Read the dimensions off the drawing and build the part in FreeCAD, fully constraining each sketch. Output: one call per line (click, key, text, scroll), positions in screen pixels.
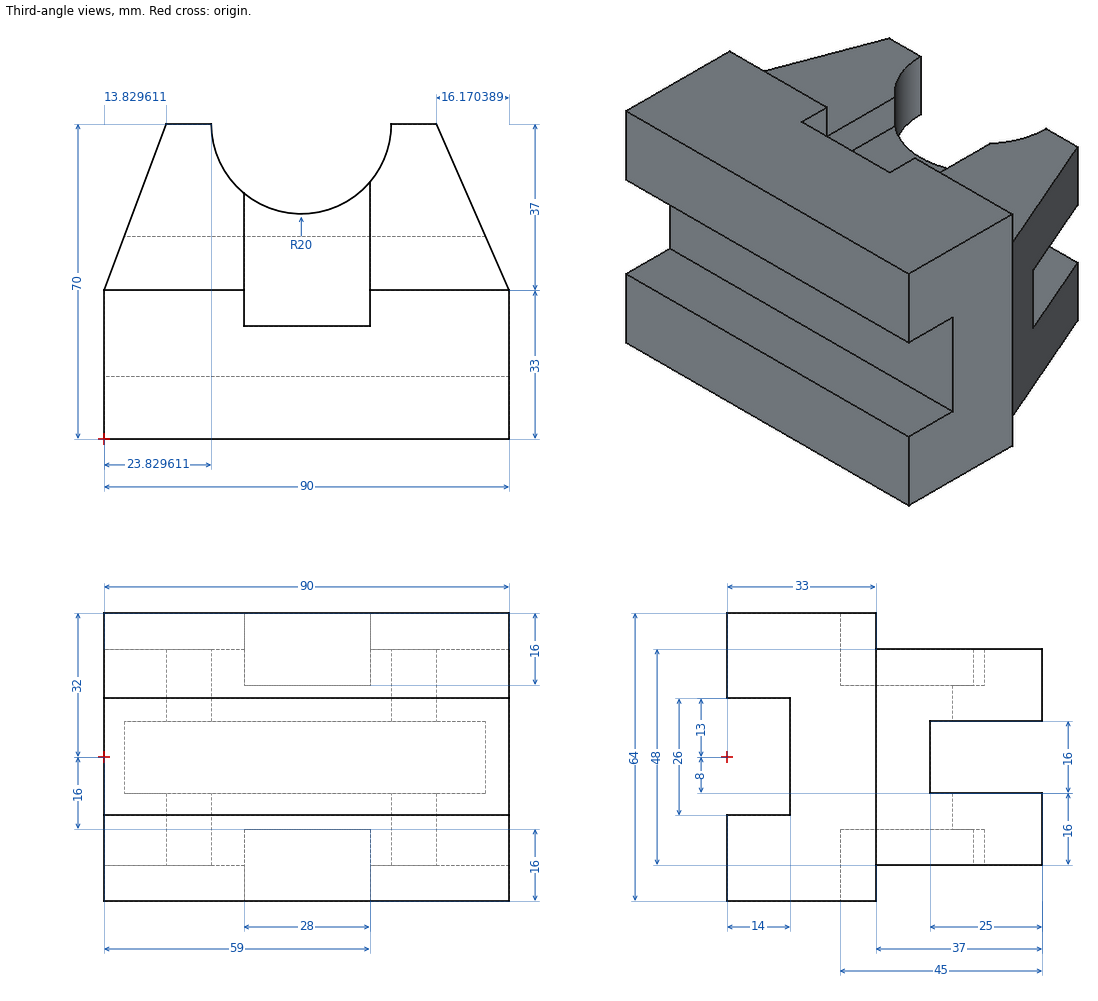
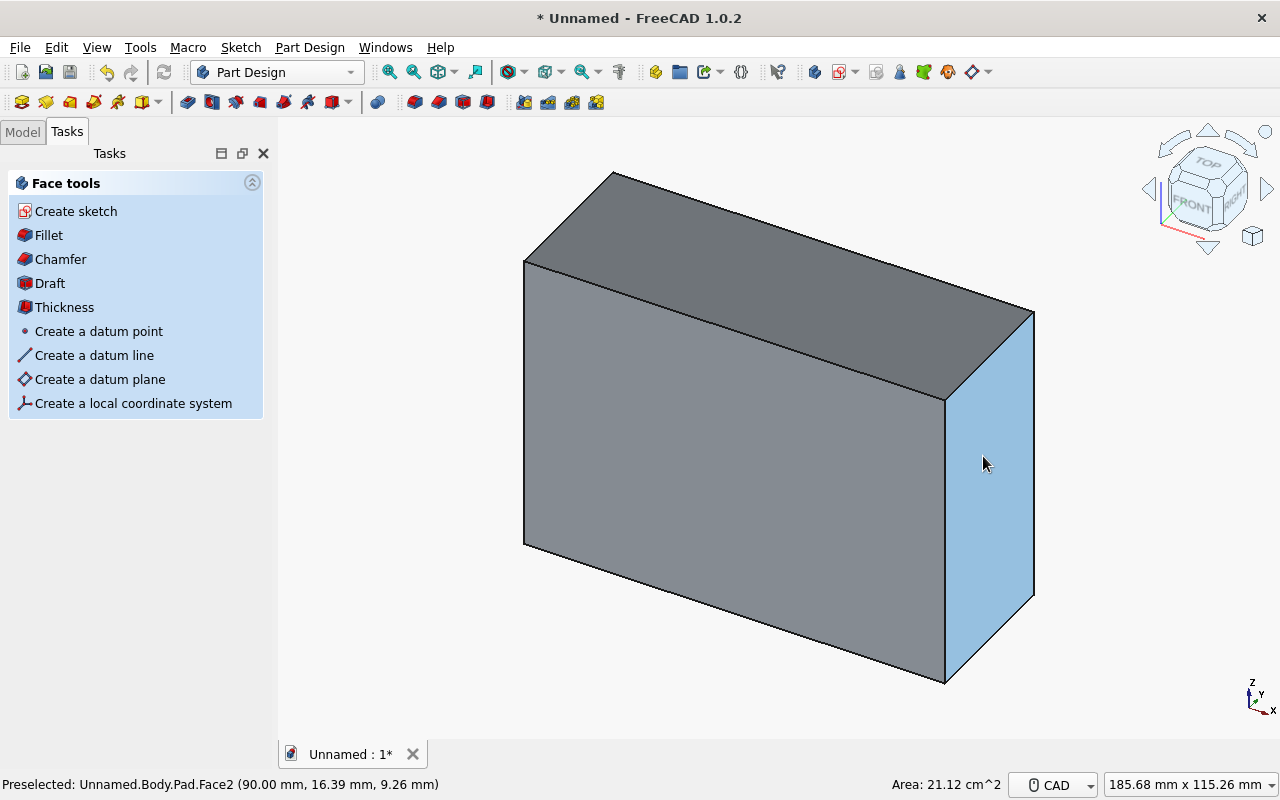
click(840, 72)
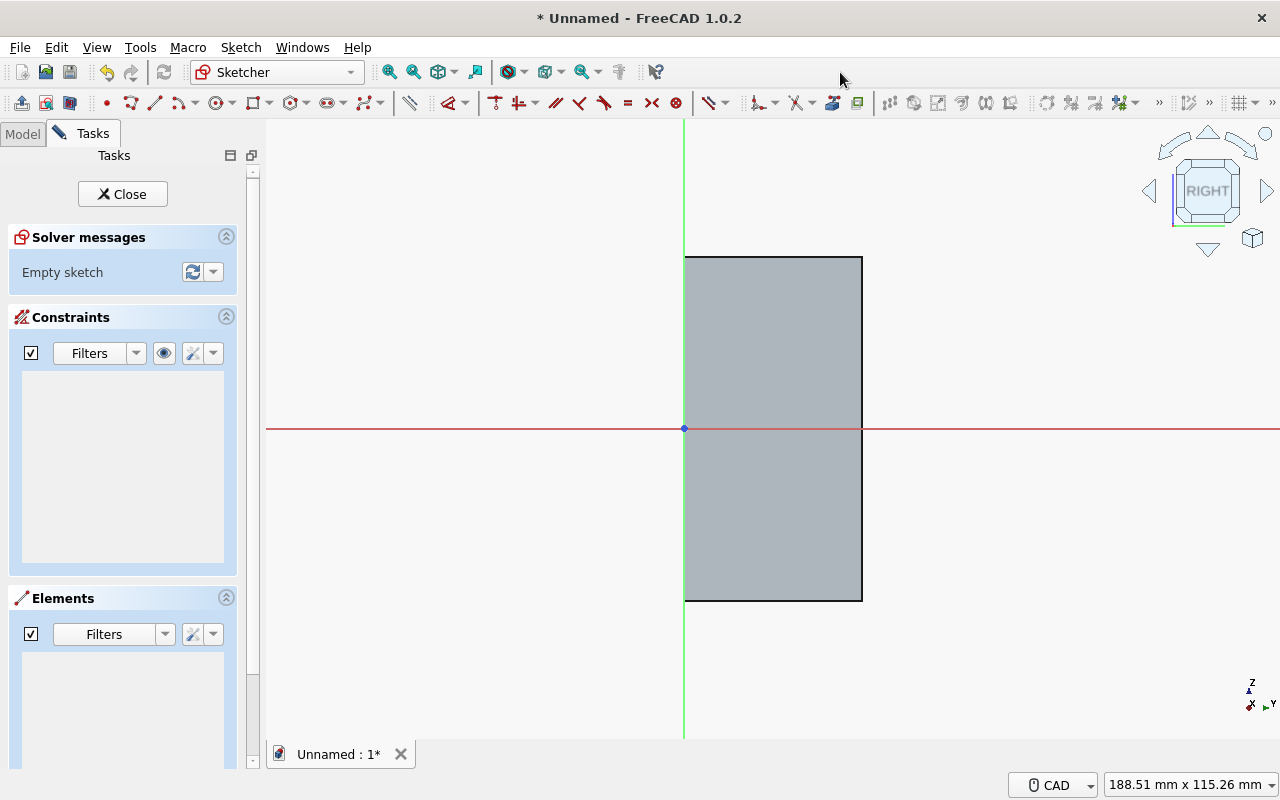
scroll(732, 429, up, 5)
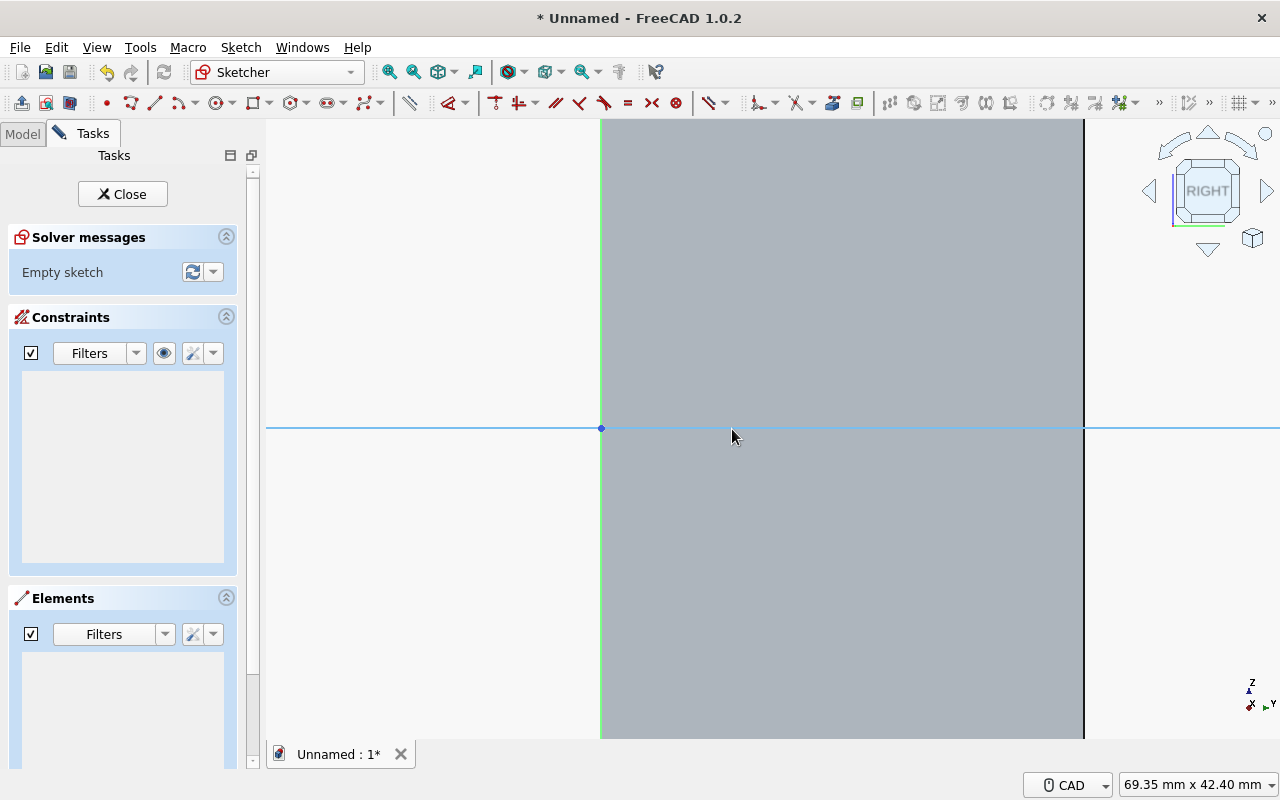
click(254, 104)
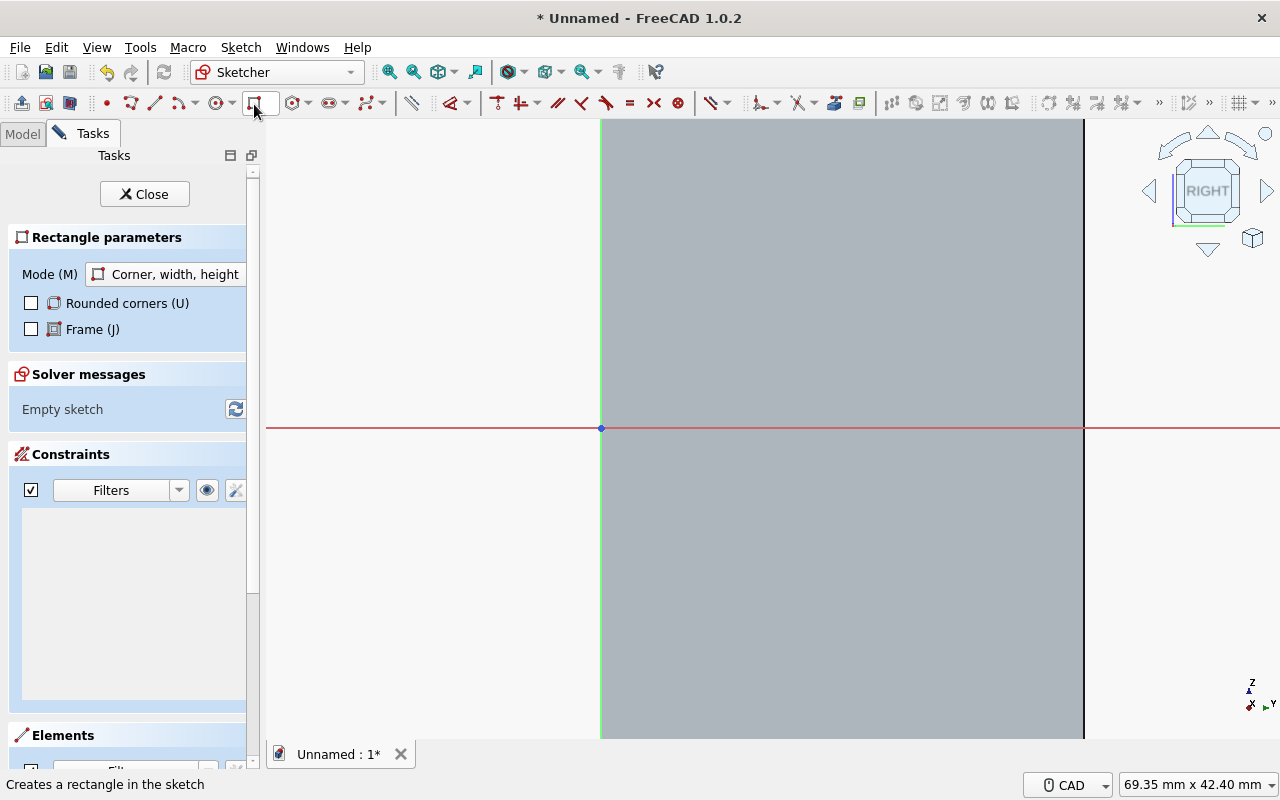
click(601, 238)
click(806, 618)
key(Escape)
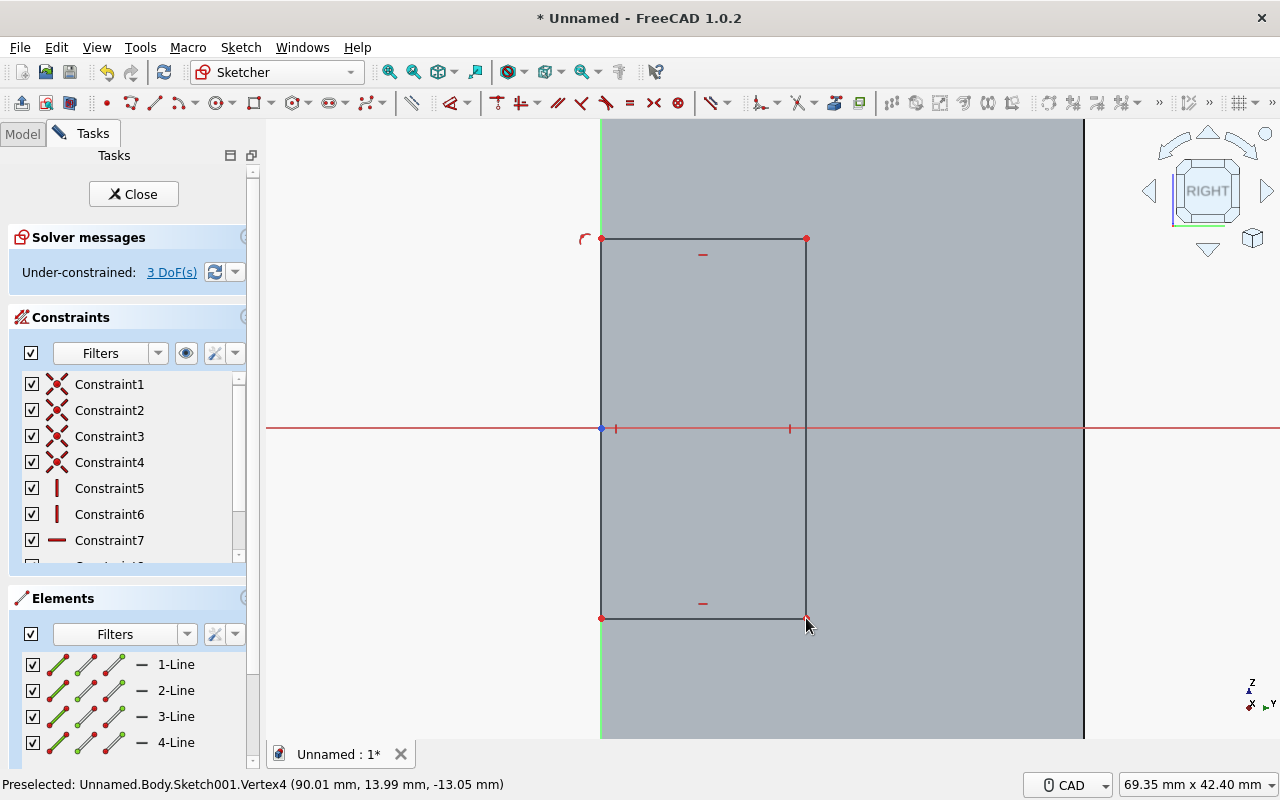
click(450, 104)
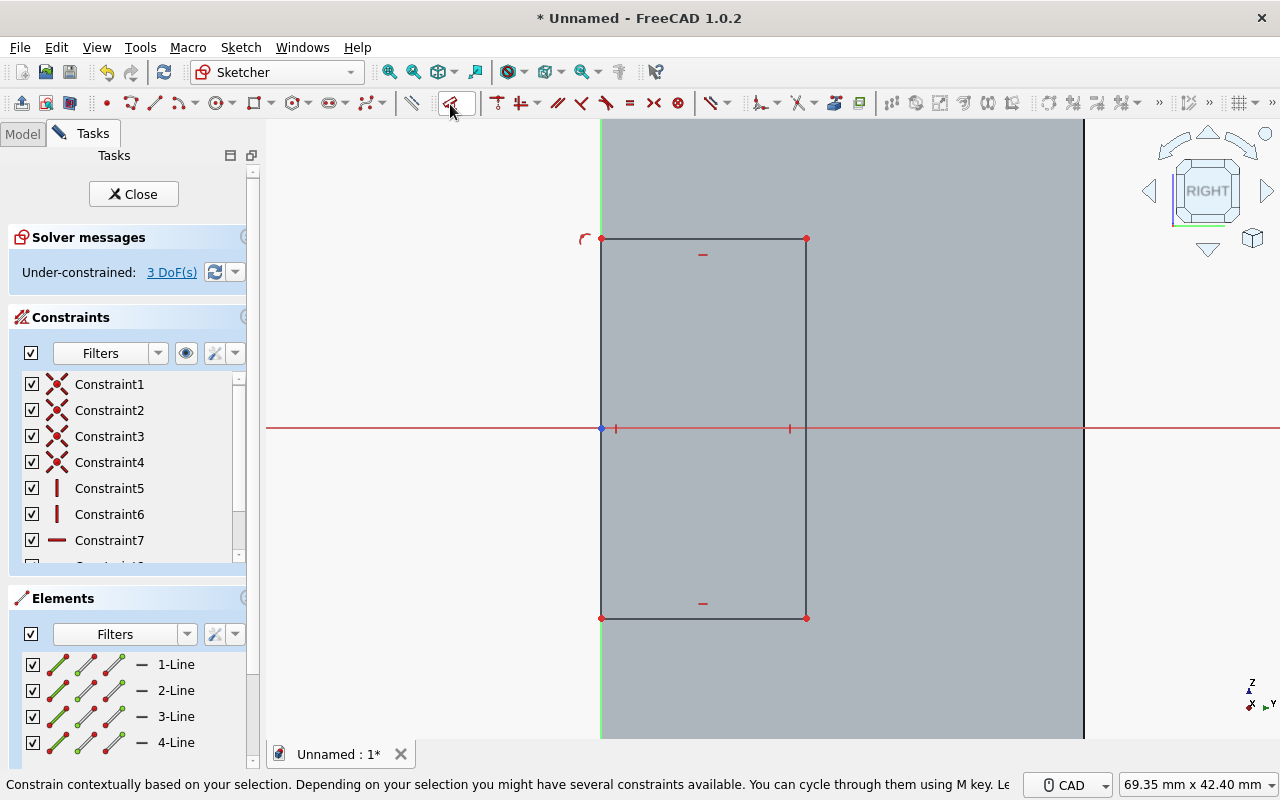
click(601, 353)
click(567, 342)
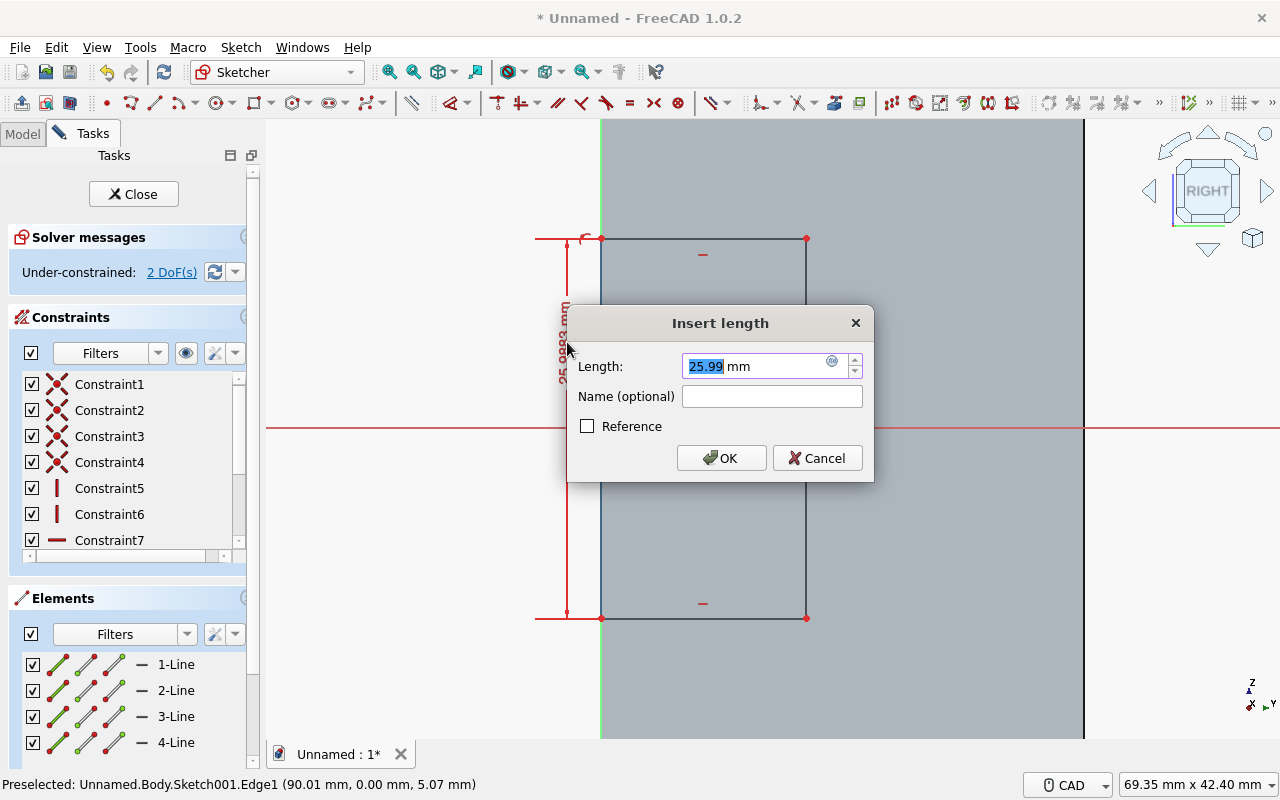
text(26)
key(Return)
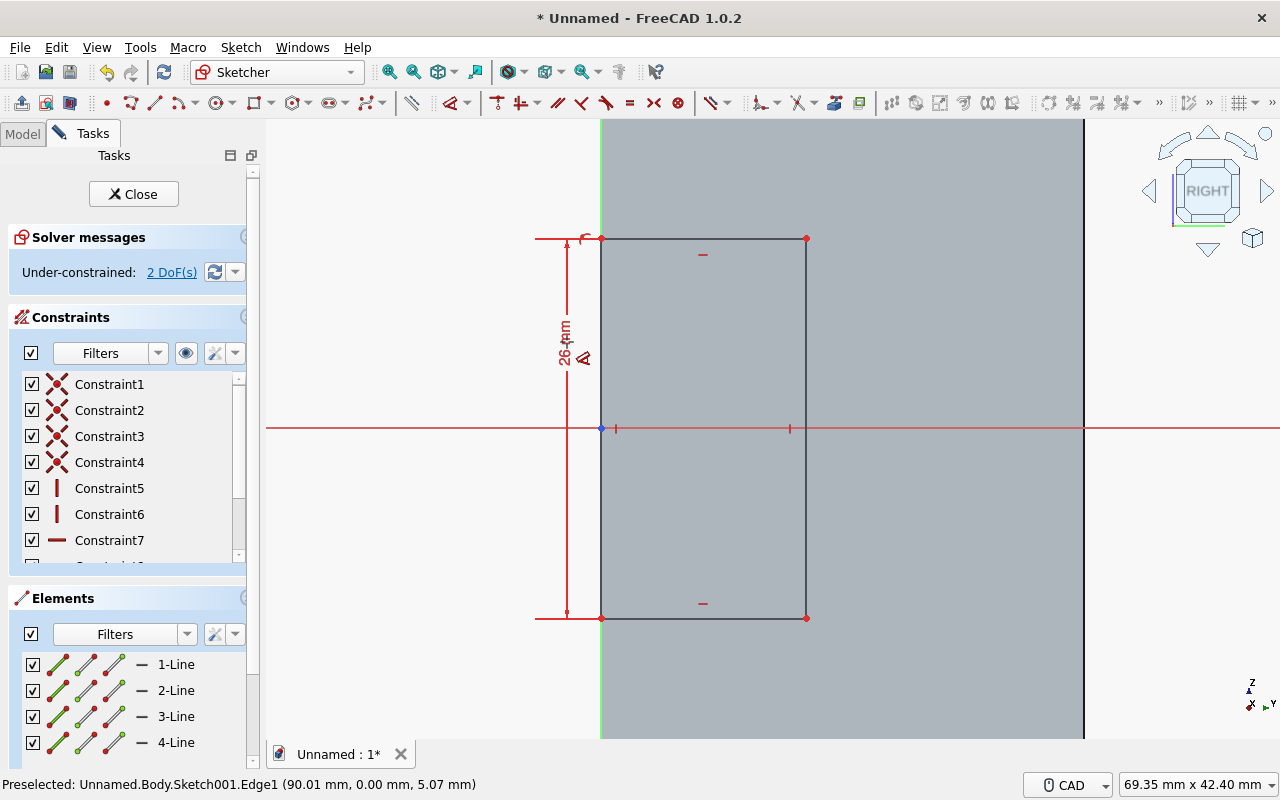
click(663, 619)
click(704, 653)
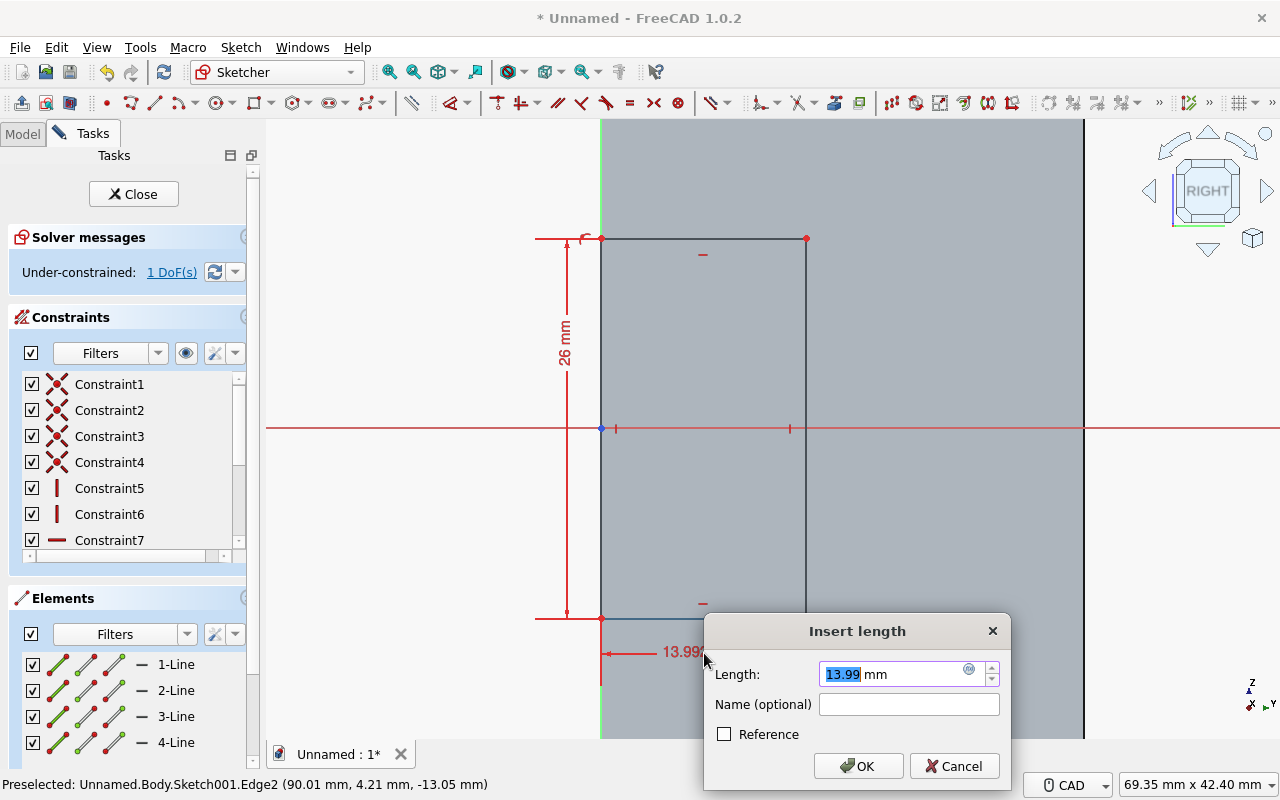
text(14)
key(Return)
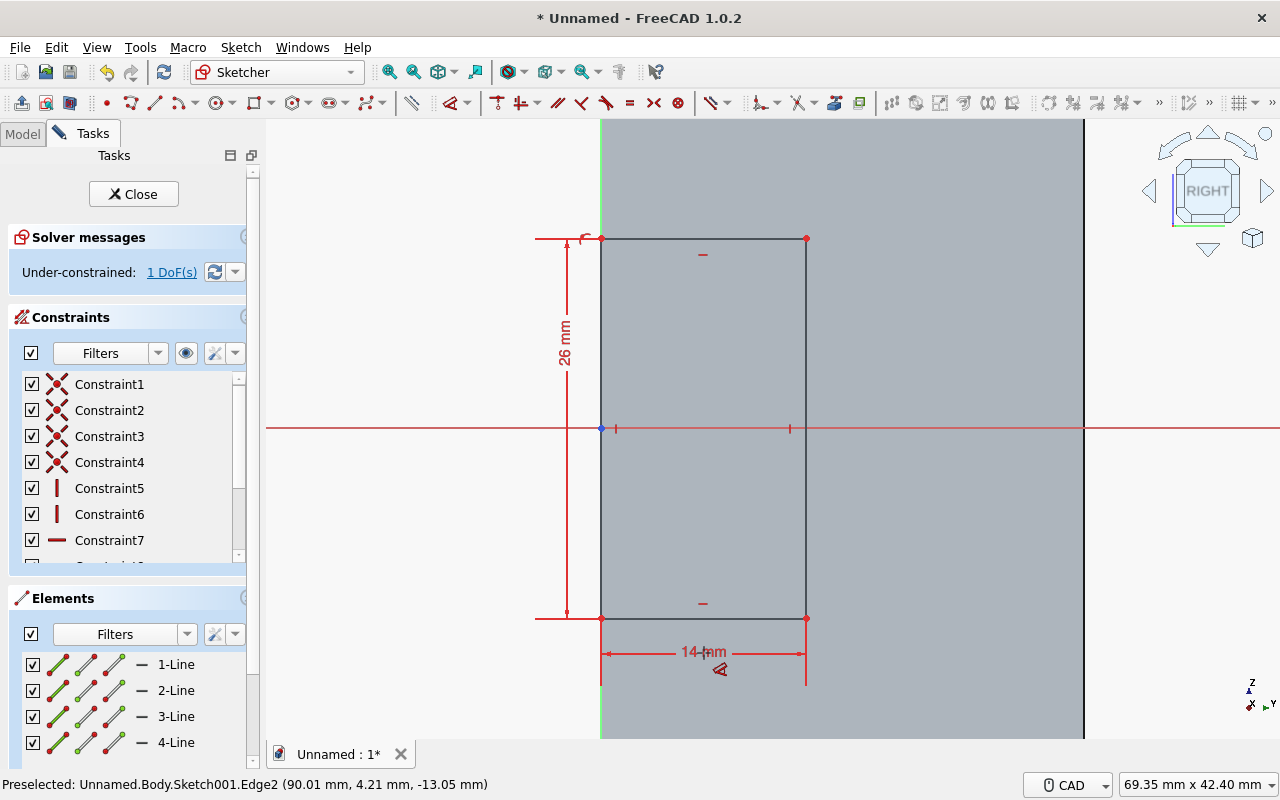
click(601, 239)
click(567, 290)